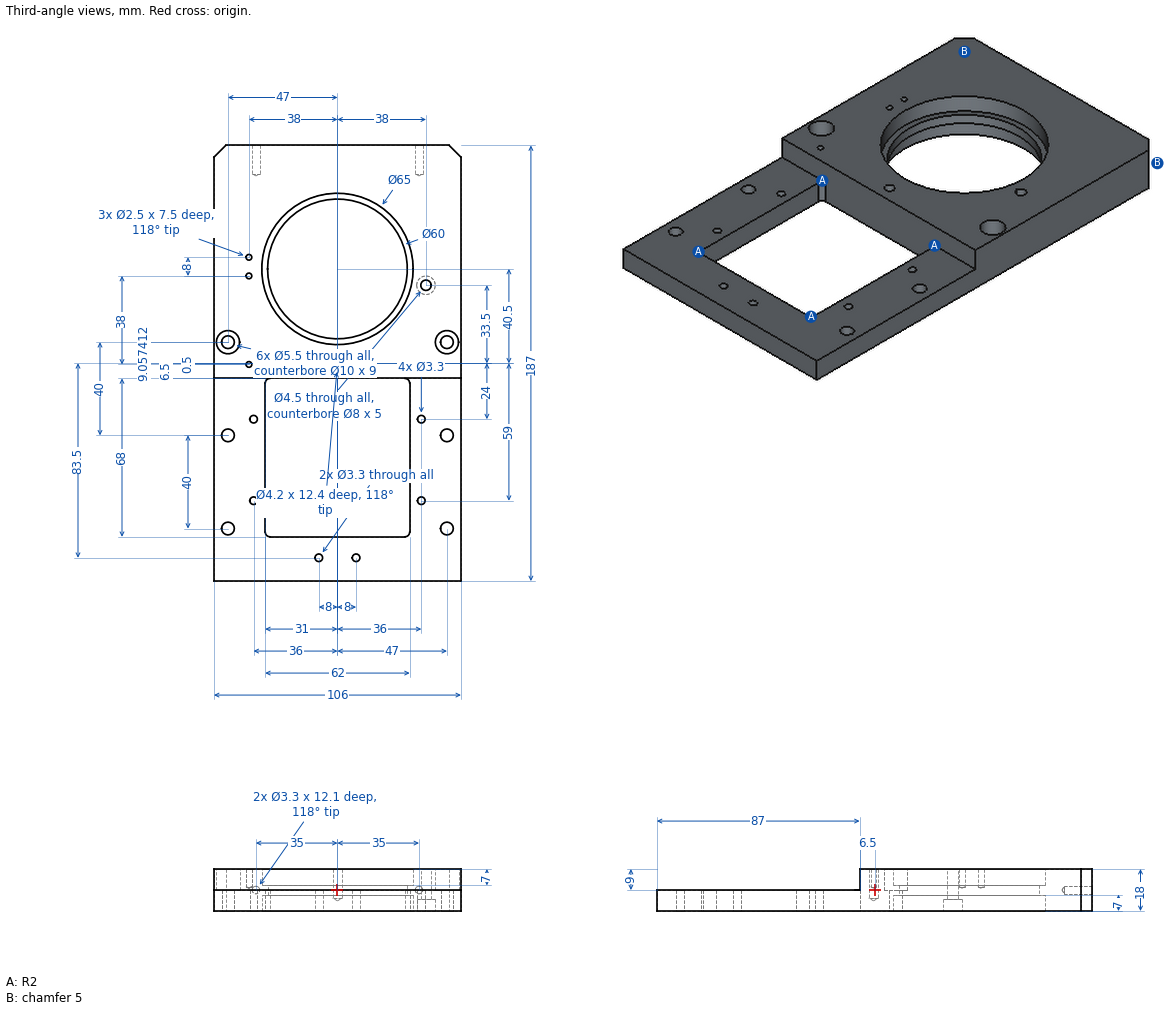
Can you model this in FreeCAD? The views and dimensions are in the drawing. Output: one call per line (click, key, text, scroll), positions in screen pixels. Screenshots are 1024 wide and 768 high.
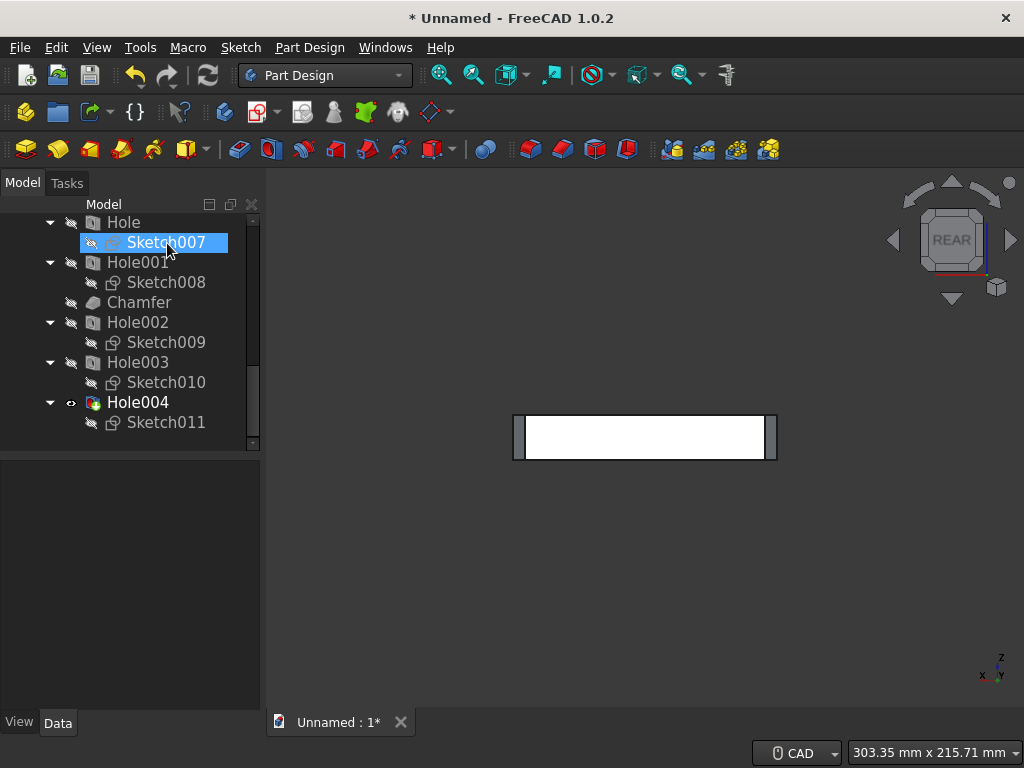
click(442, 76)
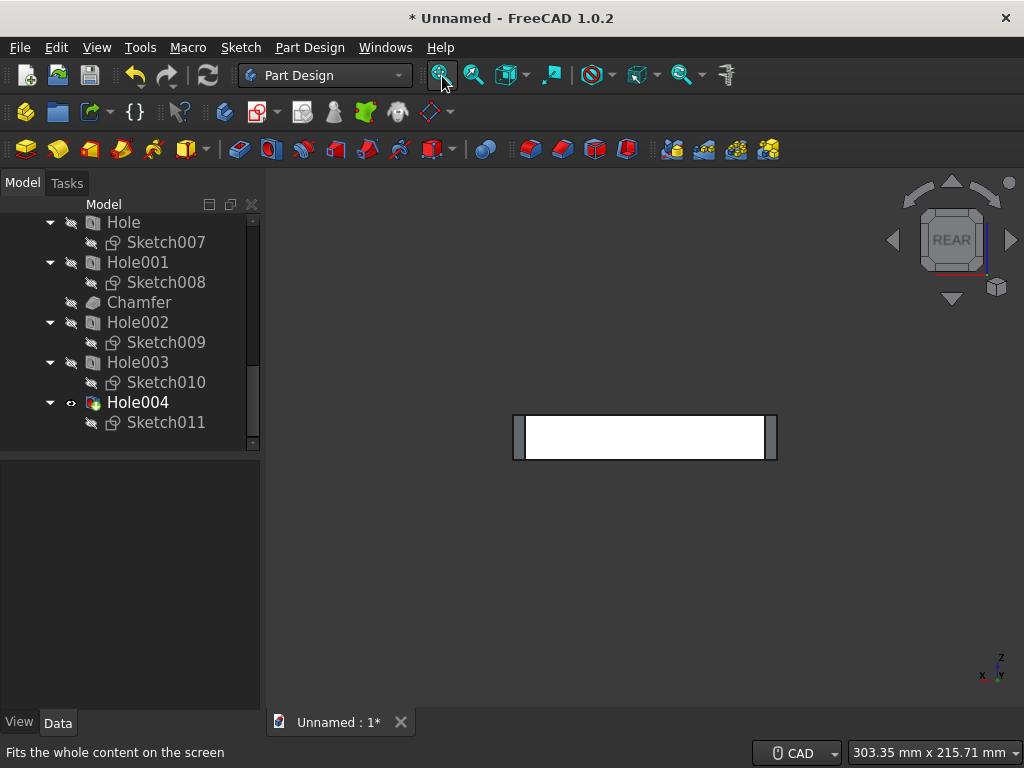
click(576, 437)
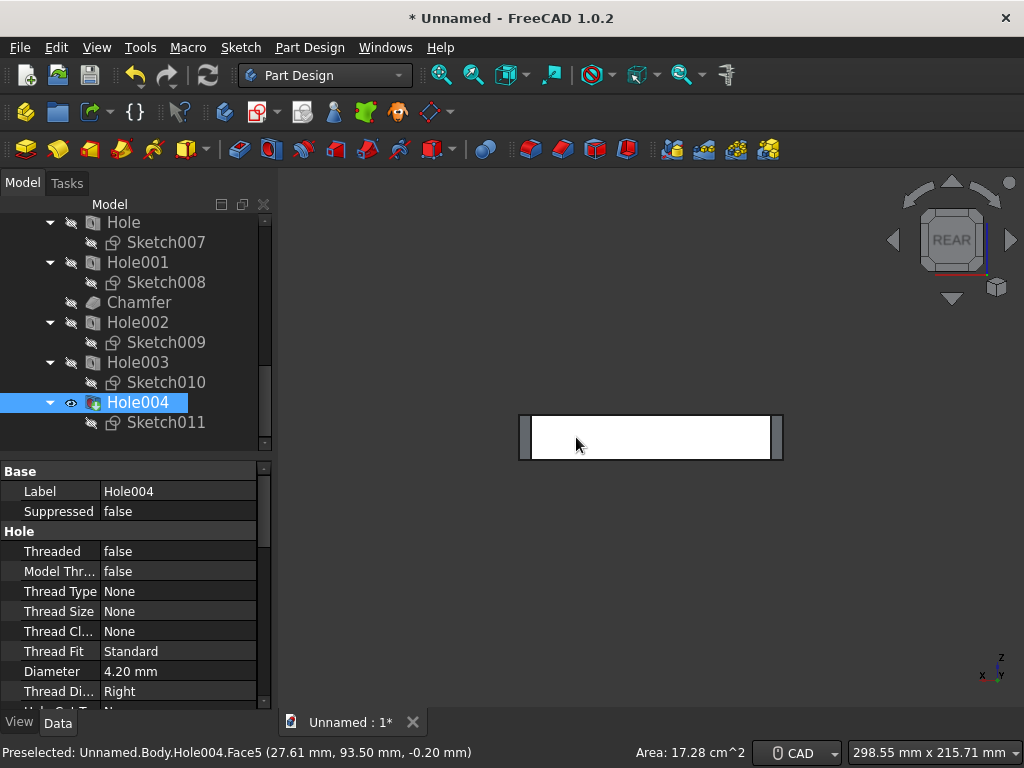
click(258, 112)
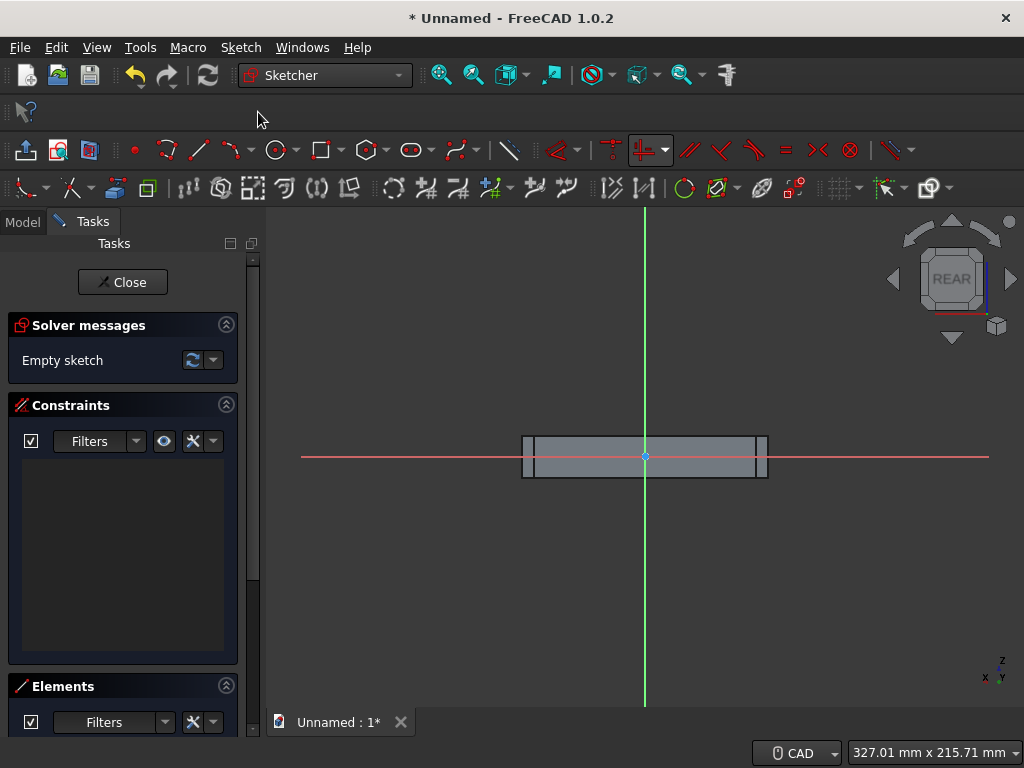
scroll(701, 457, up, 4)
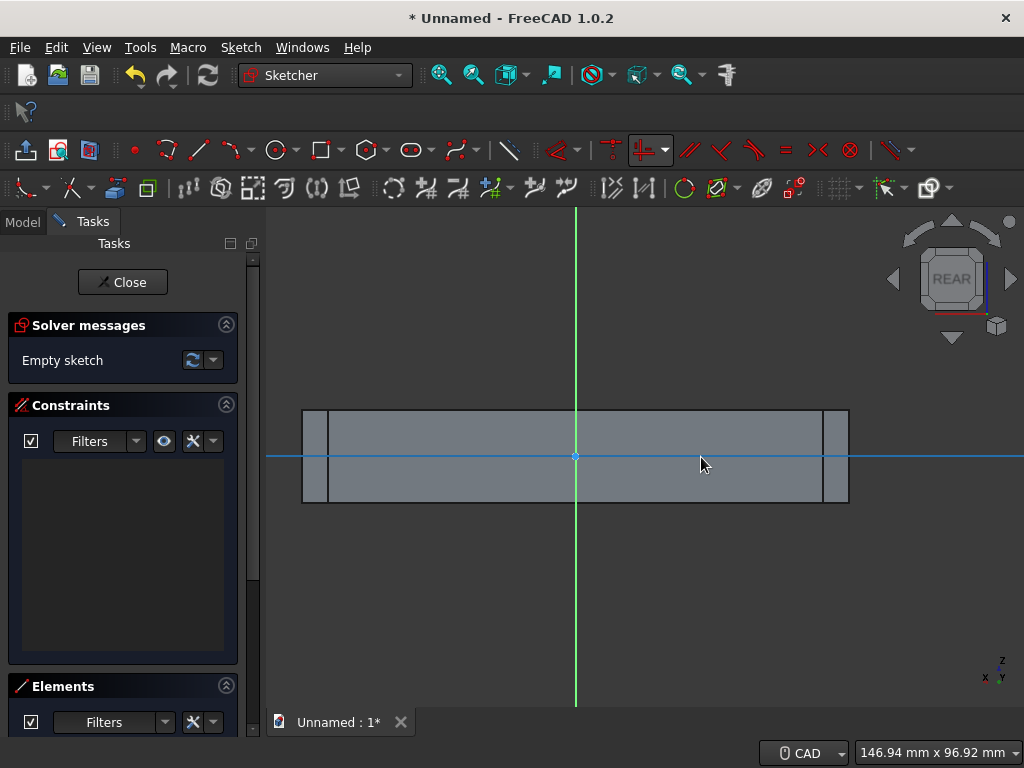
click(276, 150)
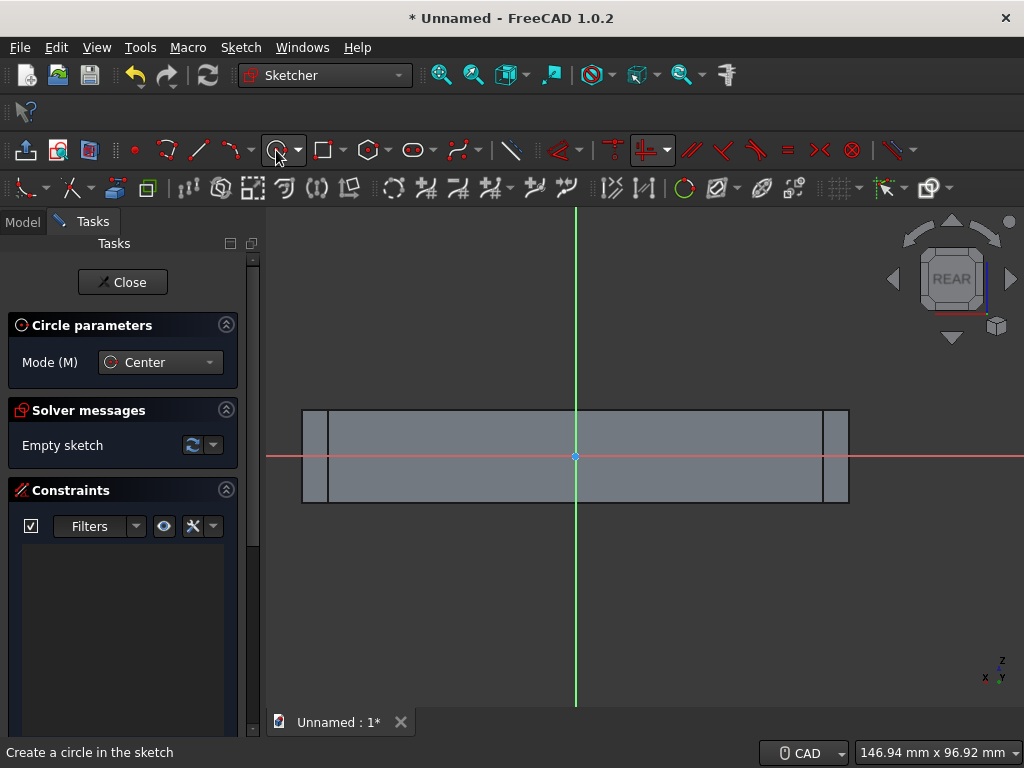
scroll(756, 456, up, 5)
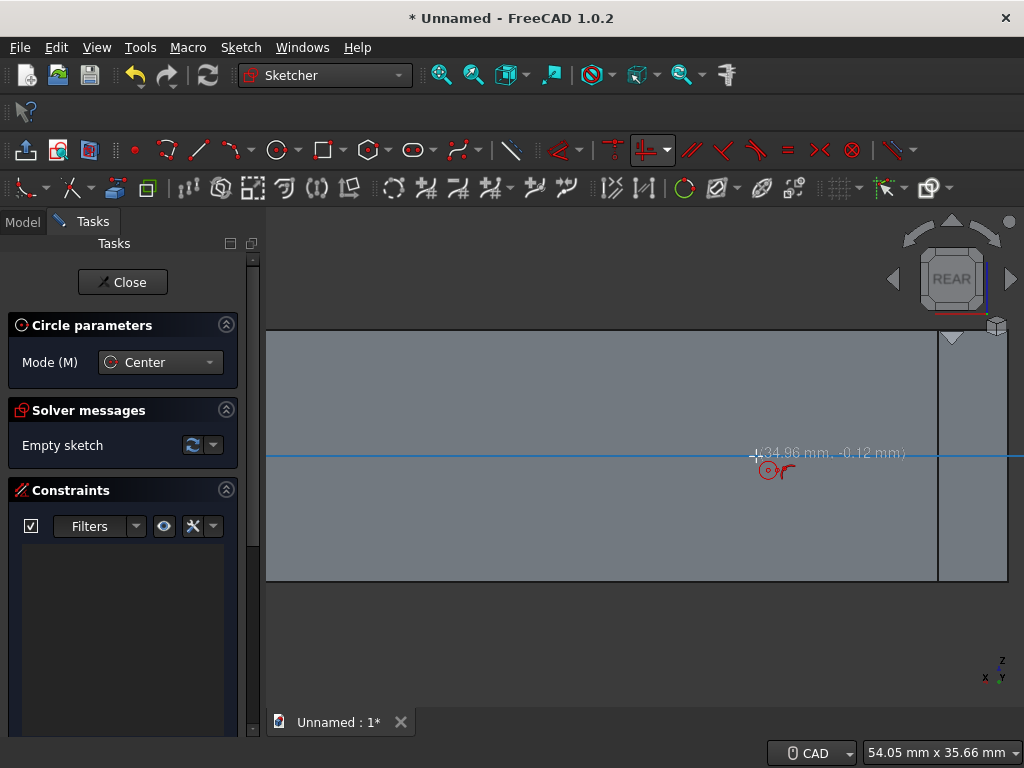
click(755, 456)
click(772, 440)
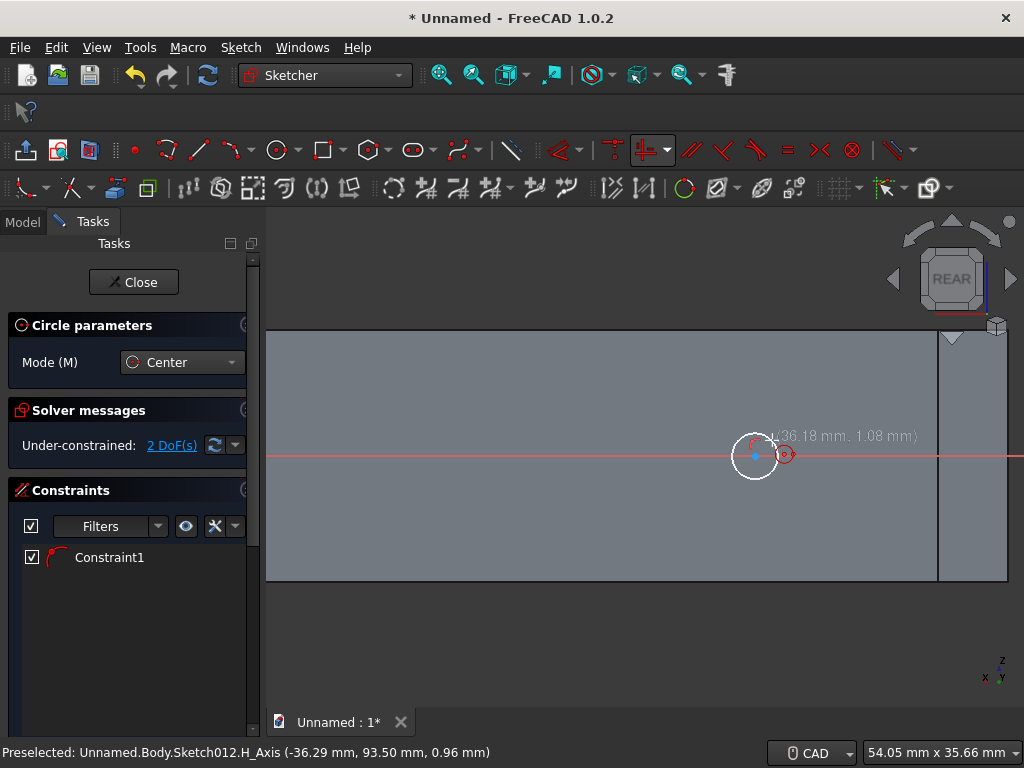
scroll(758, 457, down, 5)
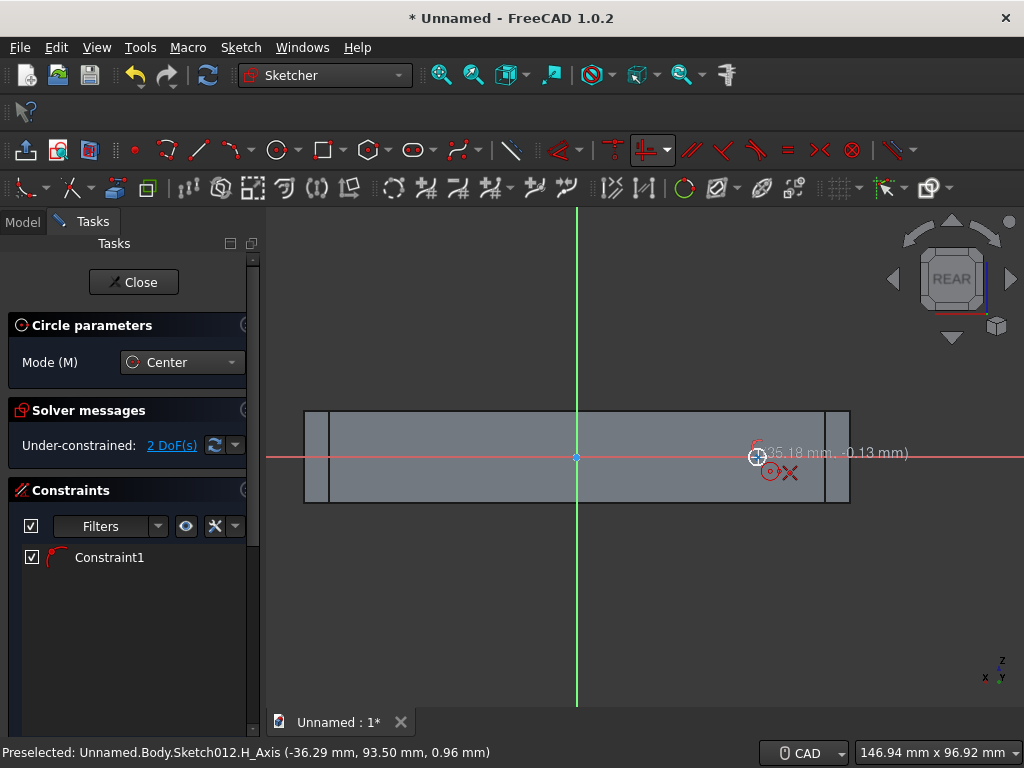
scroll(396, 457, up, 5)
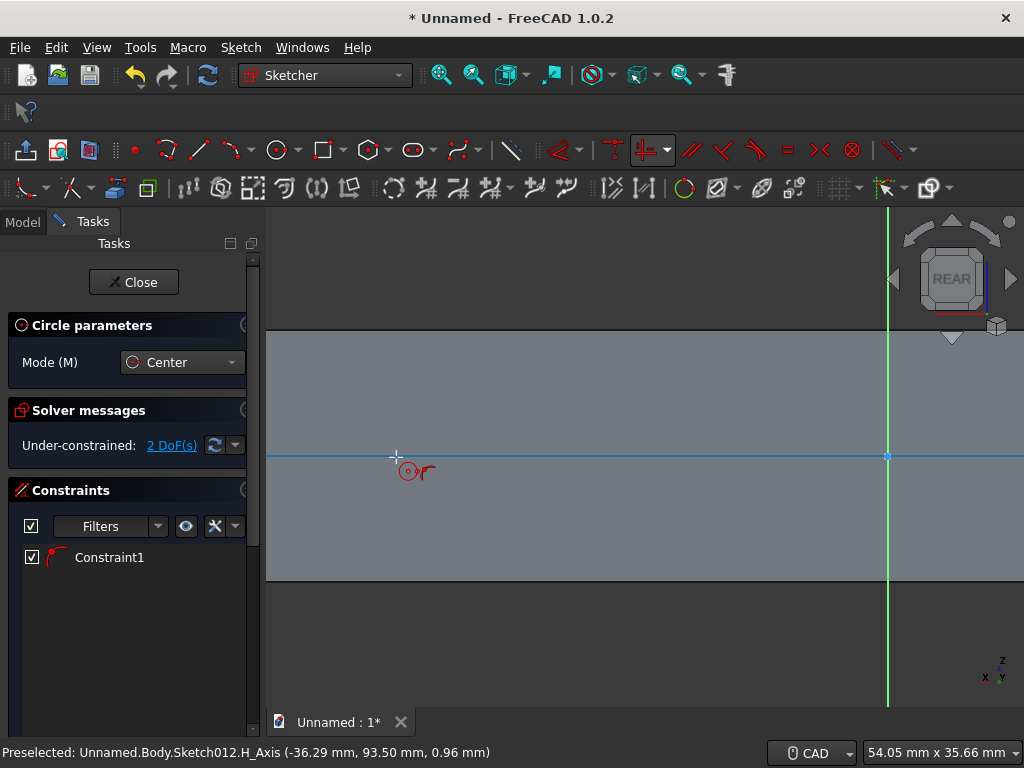
click(397, 456)
click(413, 440)
key(Escape)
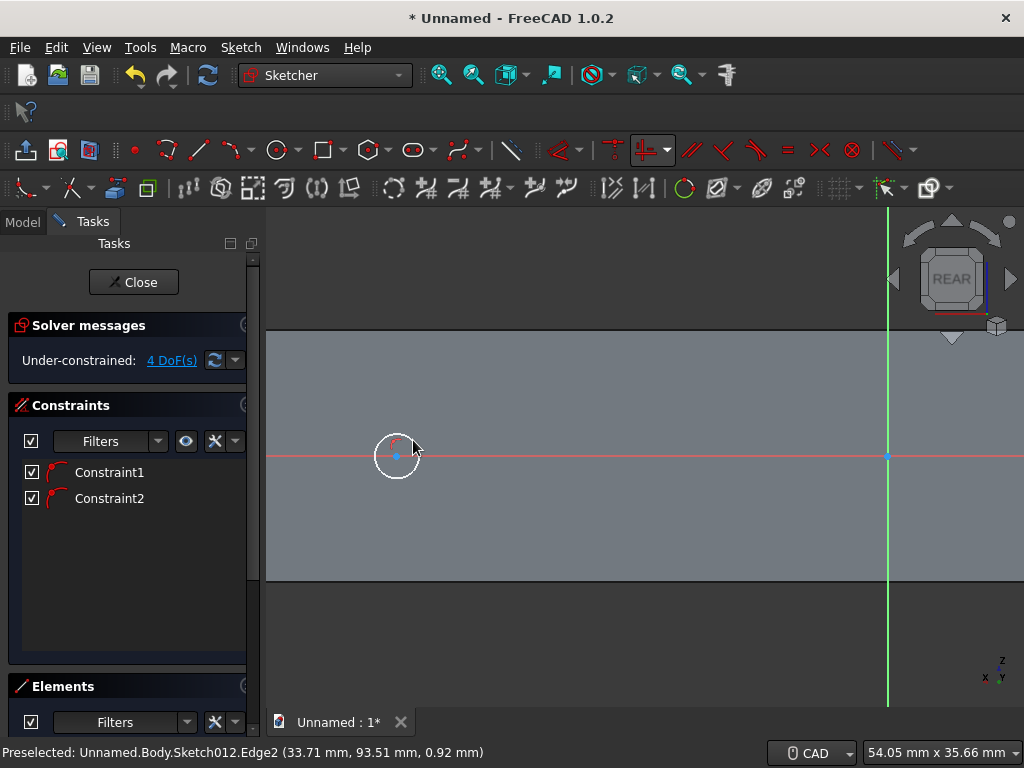
scroll(395, 457, down, 5)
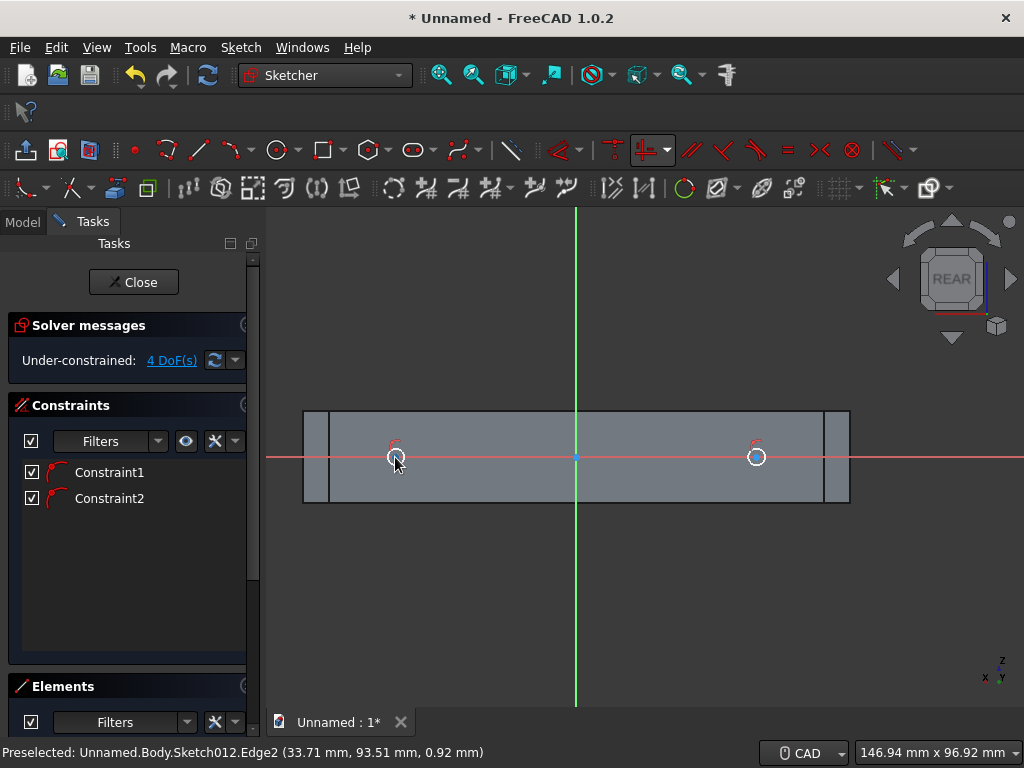
scroll(763, 451, up, 5)